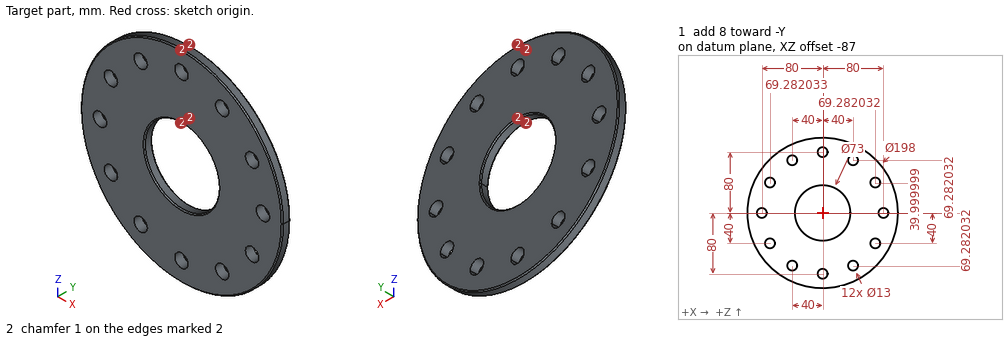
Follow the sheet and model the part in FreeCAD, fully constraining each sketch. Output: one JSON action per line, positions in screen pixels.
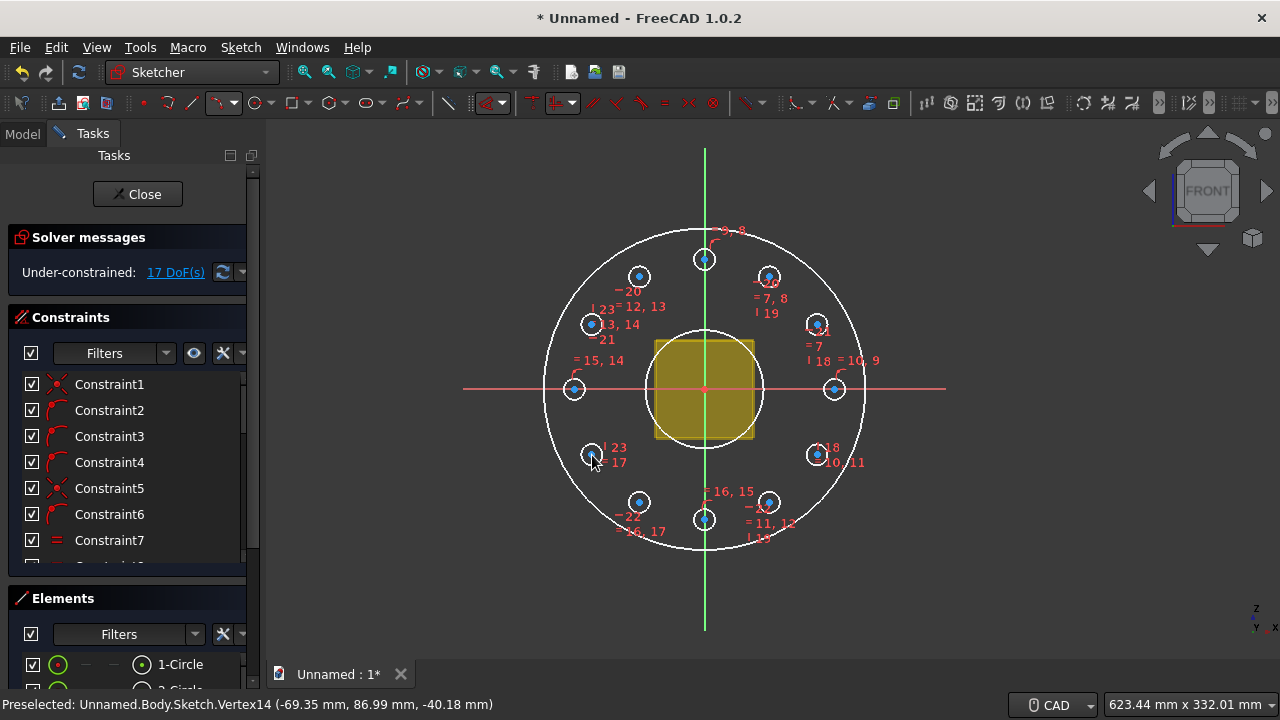
{"action": "left_click", "coordinate": [818, 275]}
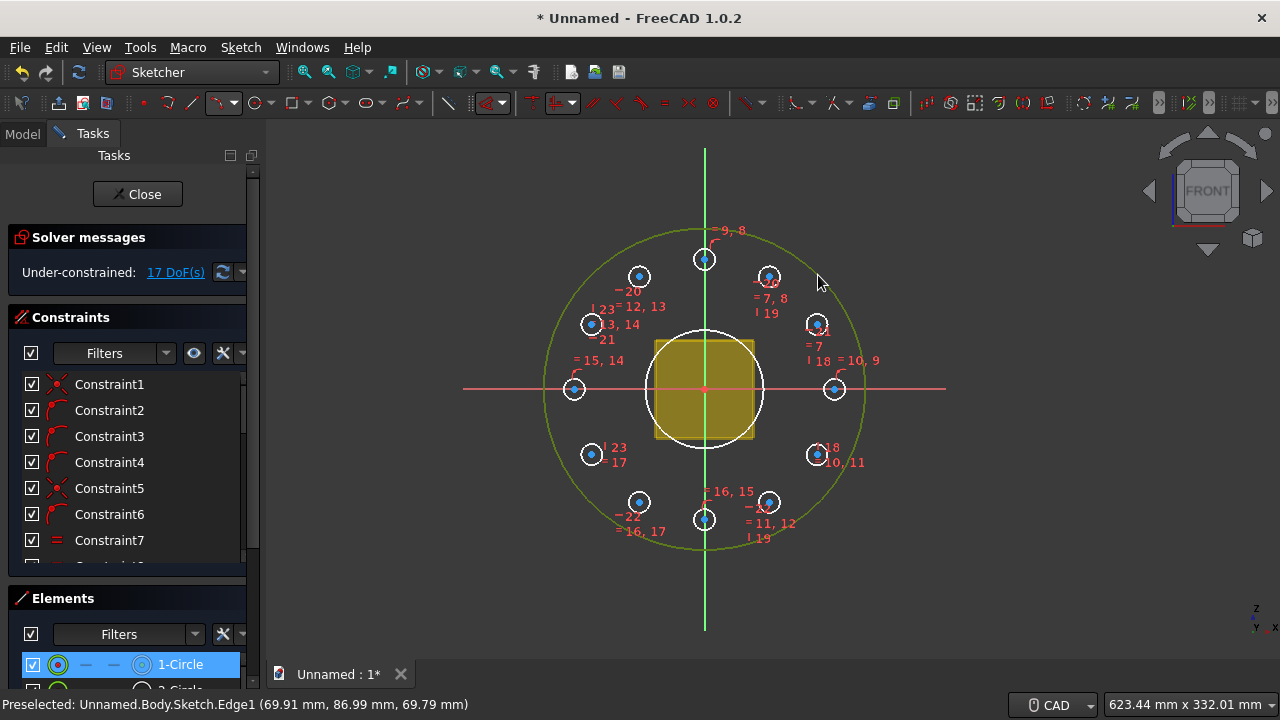
{"action": "key", "text": "k o"}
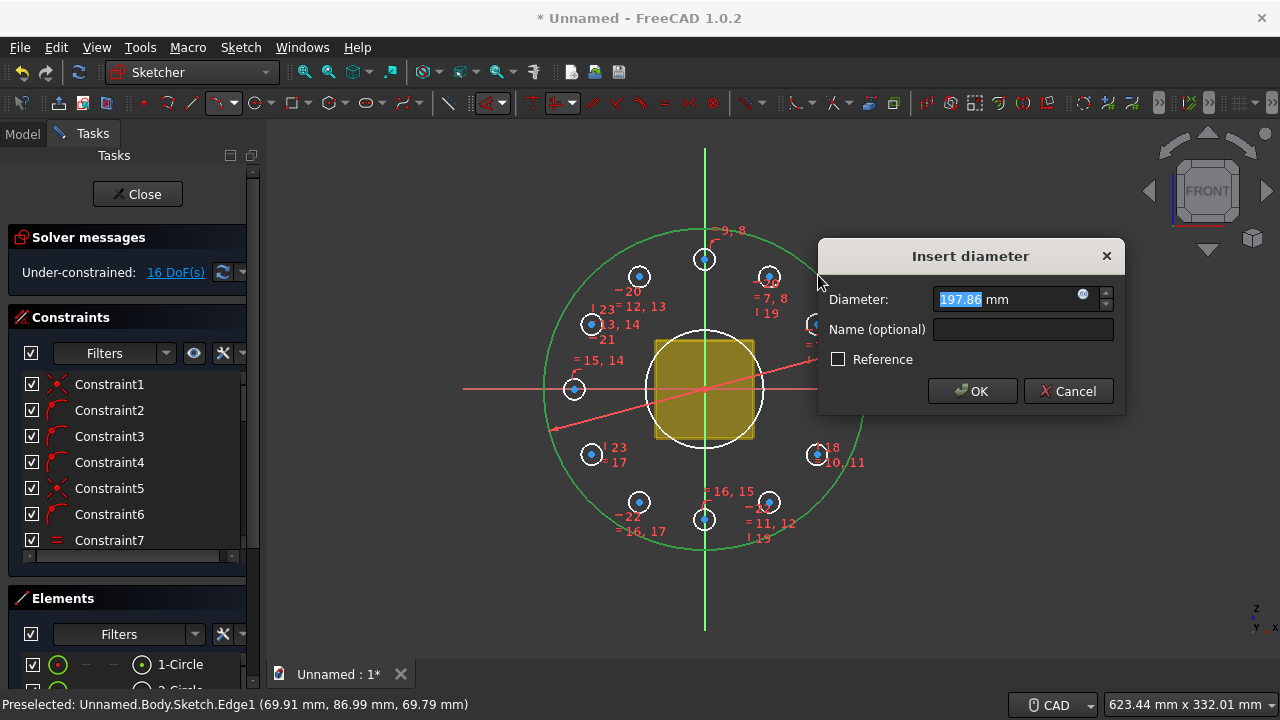
{"action": "type", "text": "198"}
{"action": "key", "text": "Return"}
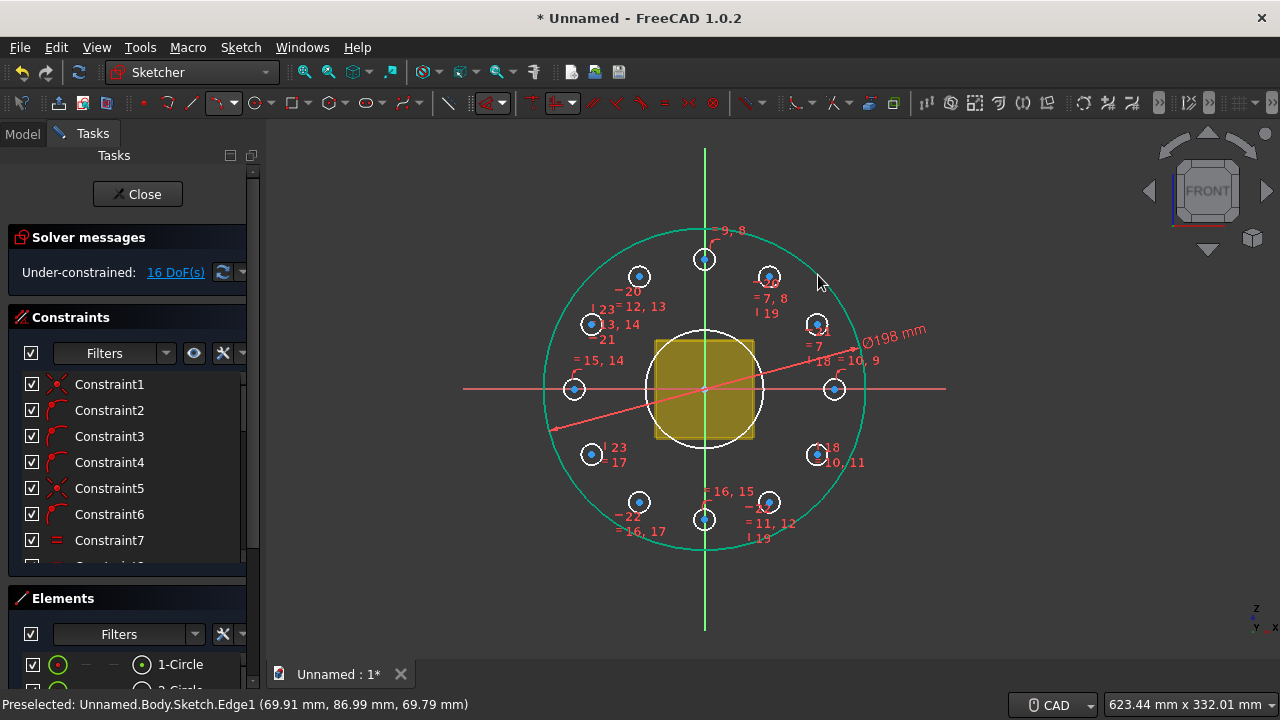
{"action": "scroll", "coordinate": [824, 317], "scroll_direction": "up", "scroll_amount": 4}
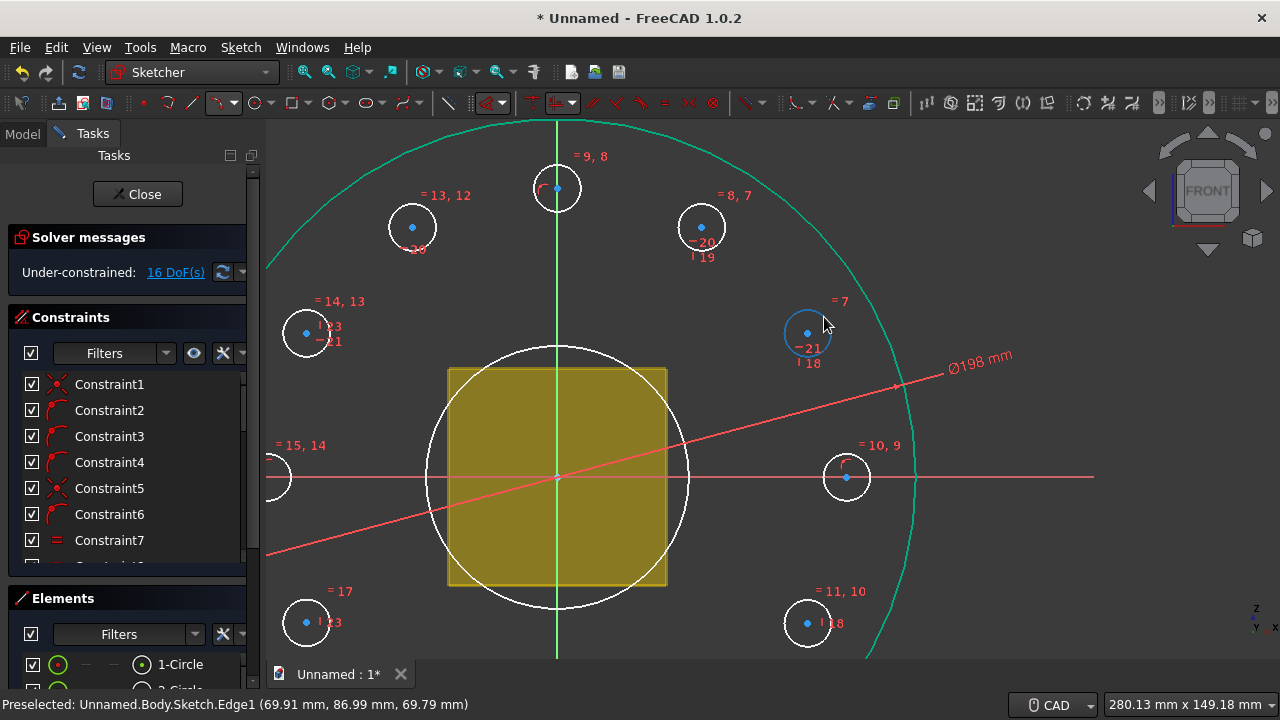
{"action": "left_click", "coordinate": [824, 317]}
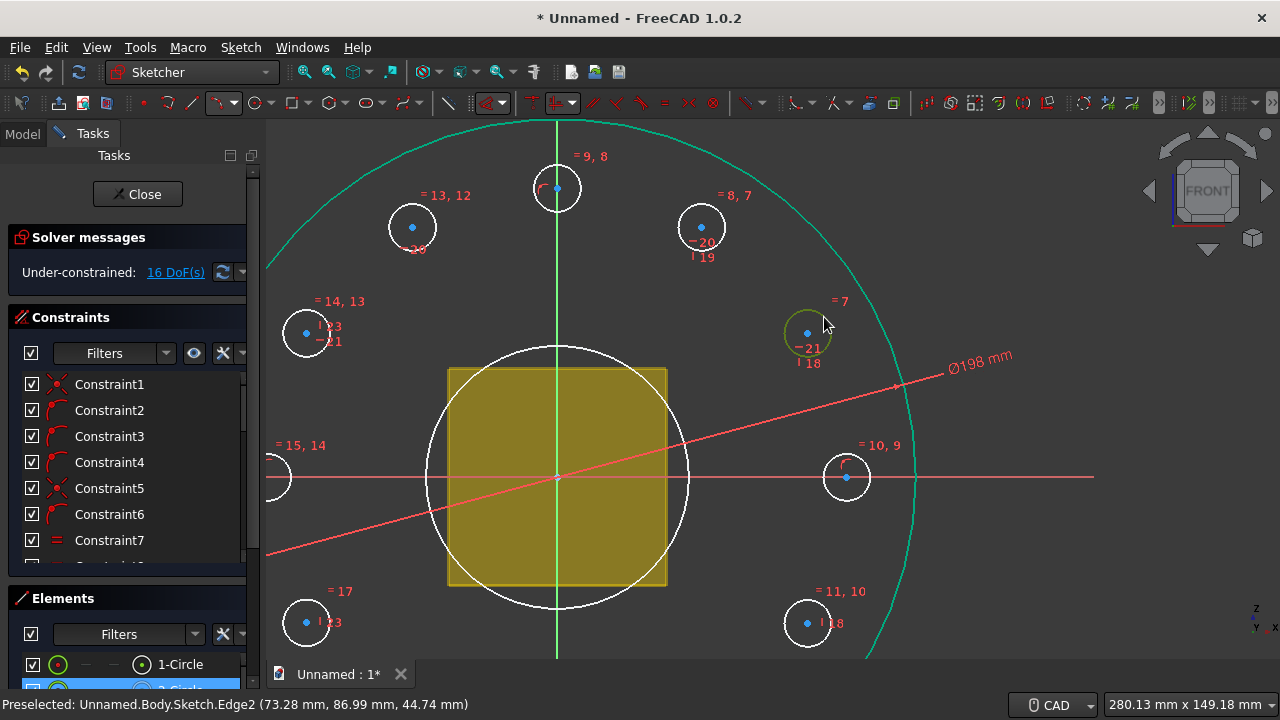
{"action": "key", "text": "k o"}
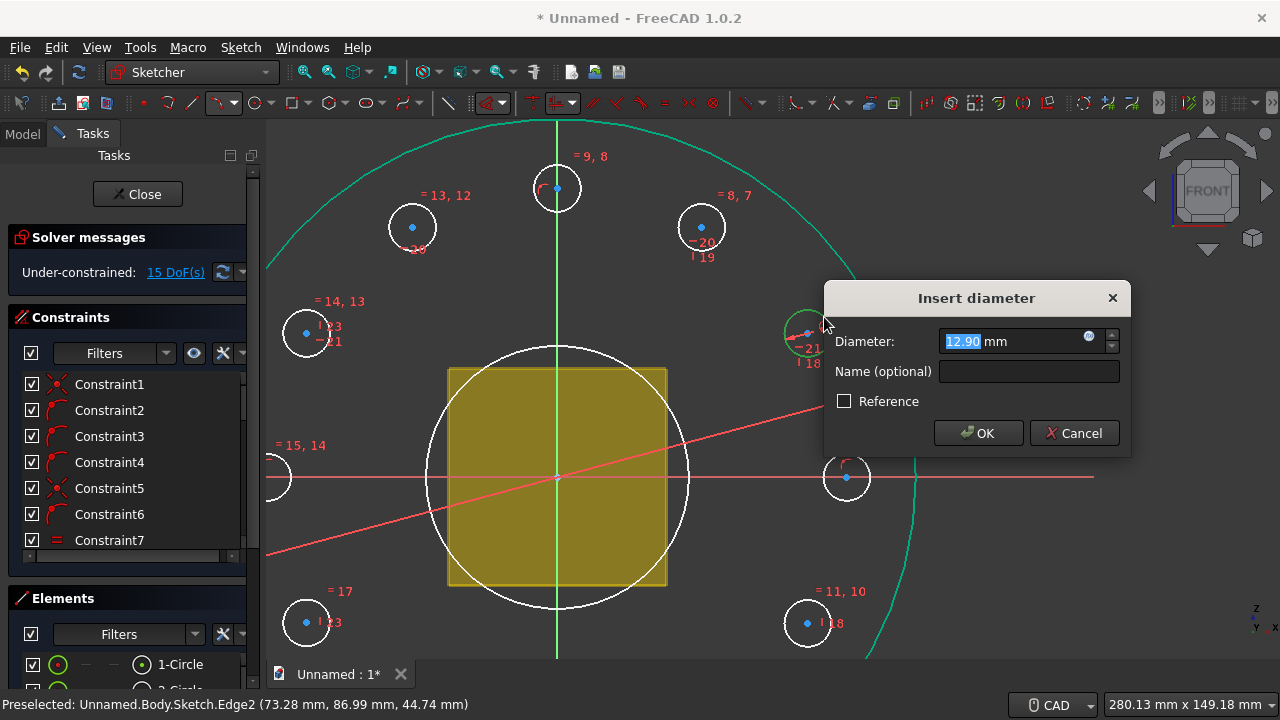
{"action": "type", "text": "13"}
{"action": "key", "text": "Return"}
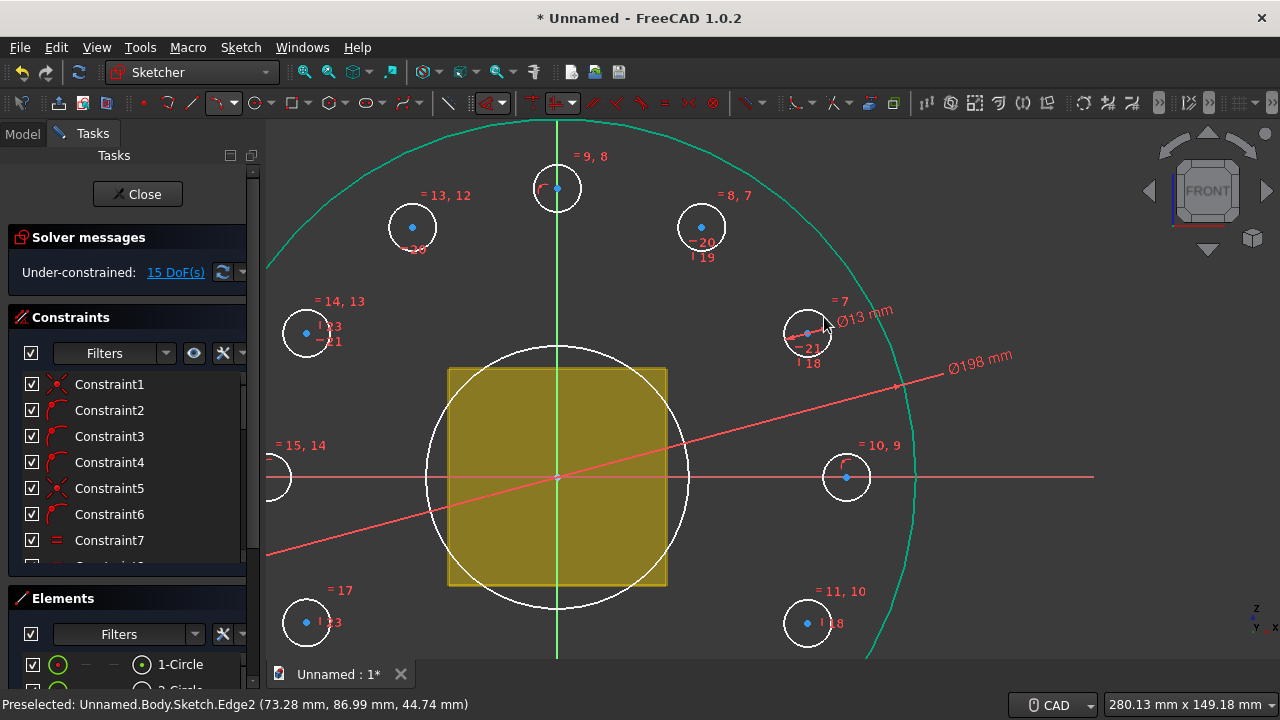
{"action": "left_click", "coordinate": [650, 384]}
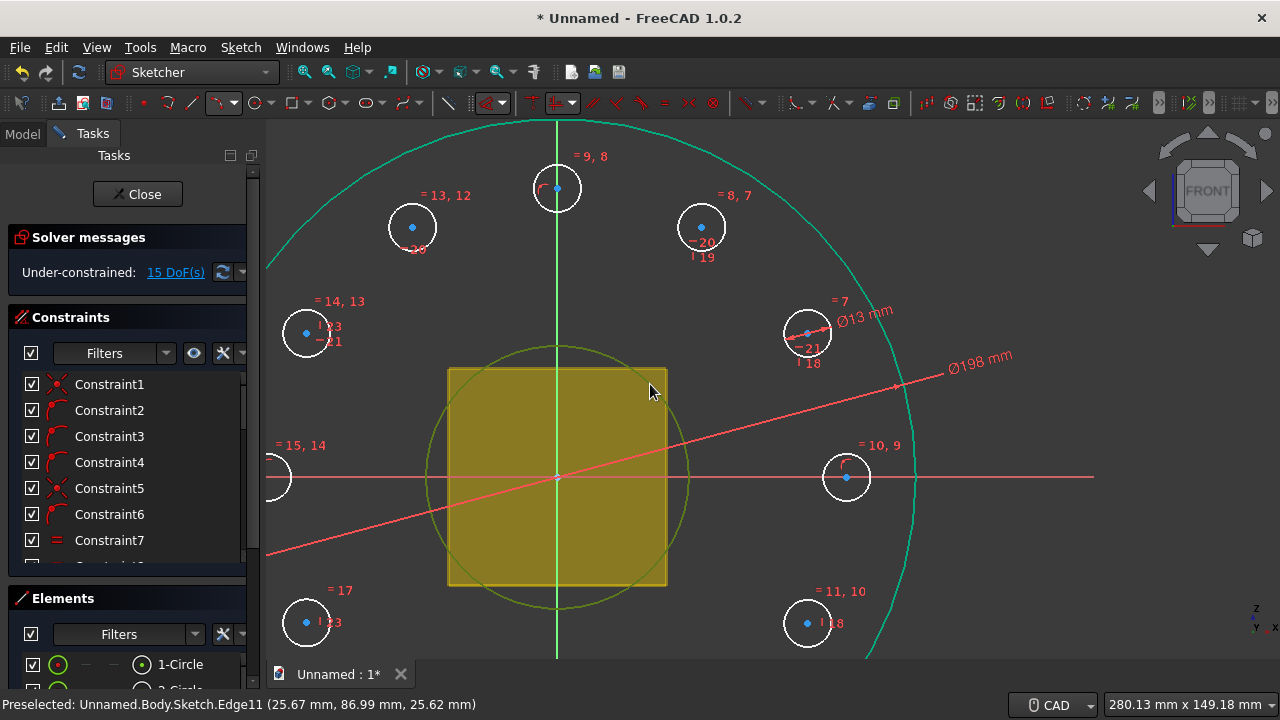
{"action": "key", "text": "k o"}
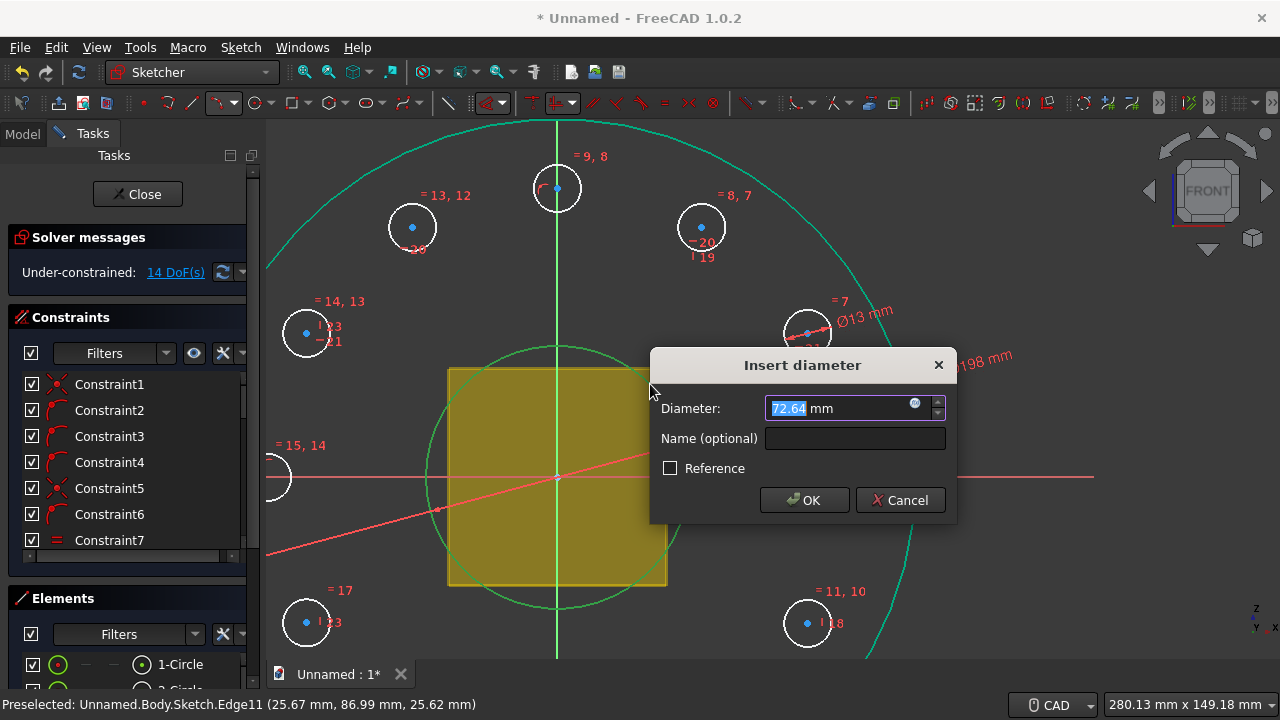
{"action": "type", "text": "73"}
{"action": "key", "text": "Return"}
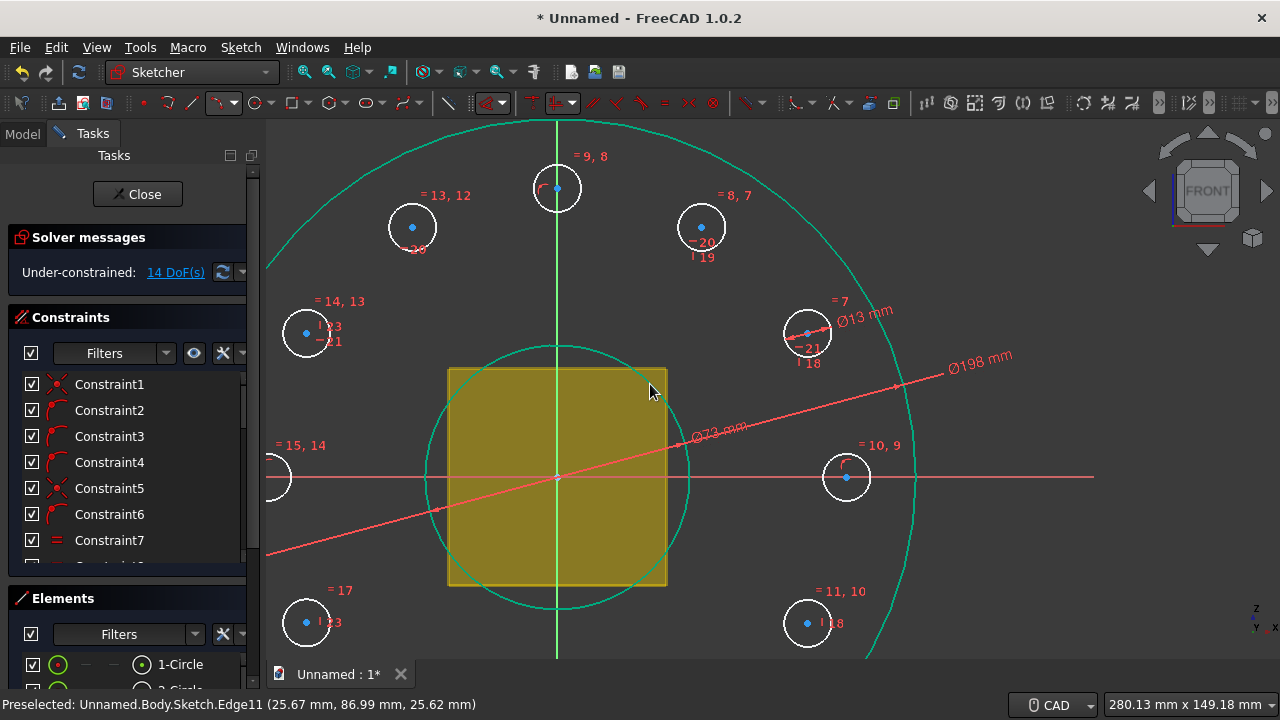
{"action": "left_click", "coordinate": [702, 227]}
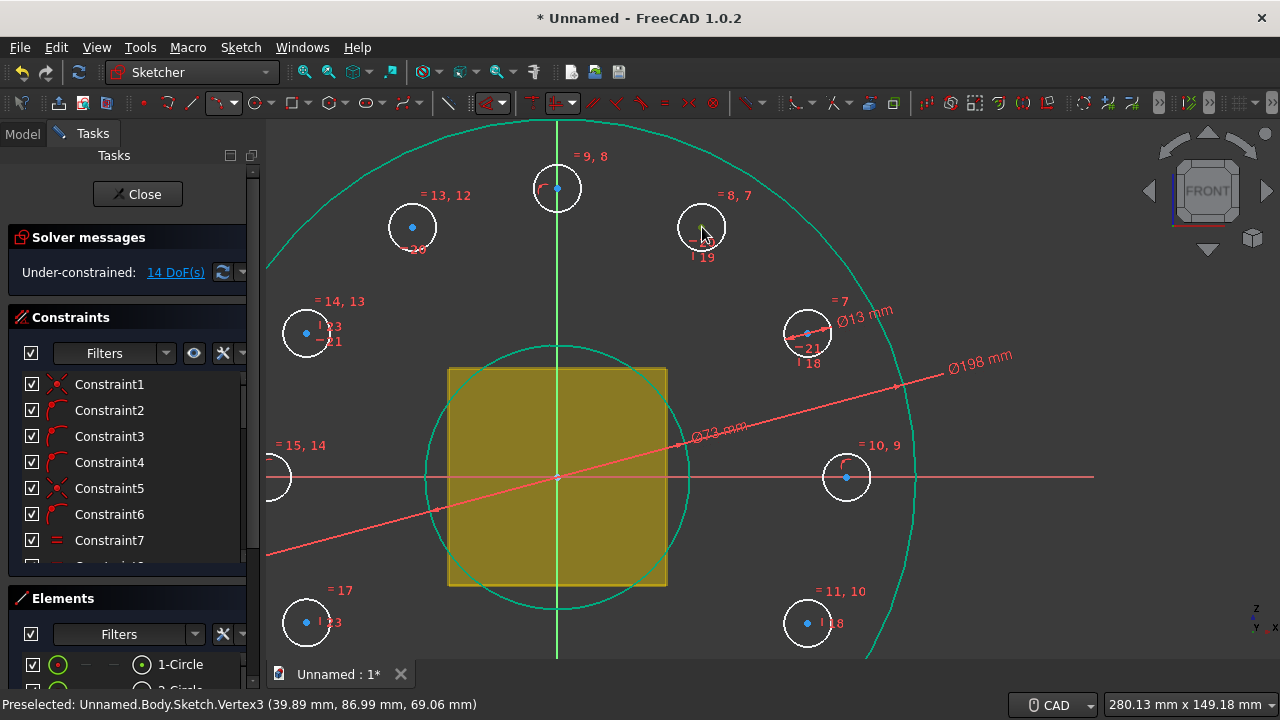
{"action": "key", "text": "l"}